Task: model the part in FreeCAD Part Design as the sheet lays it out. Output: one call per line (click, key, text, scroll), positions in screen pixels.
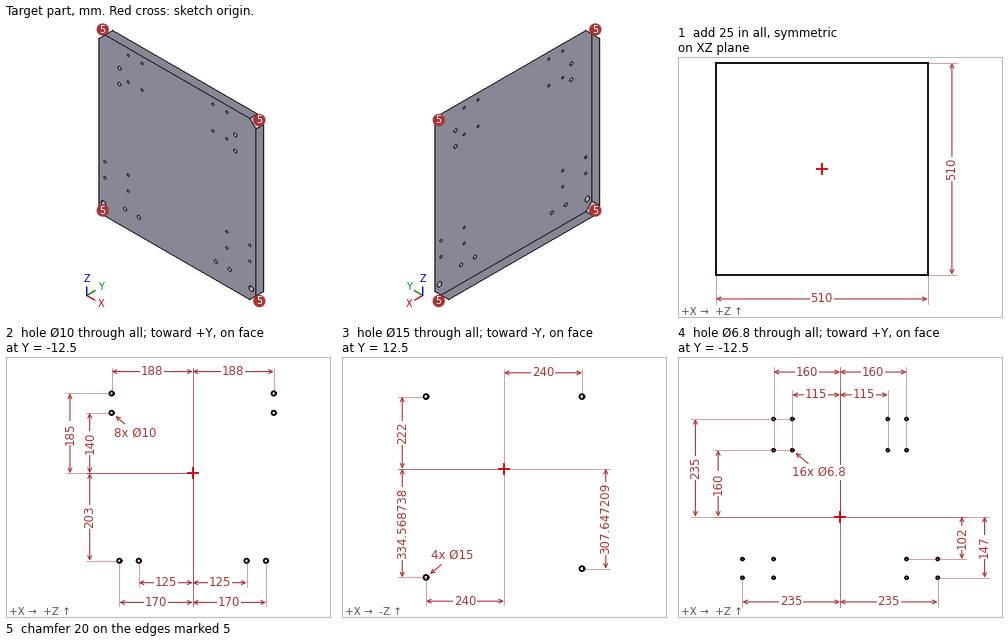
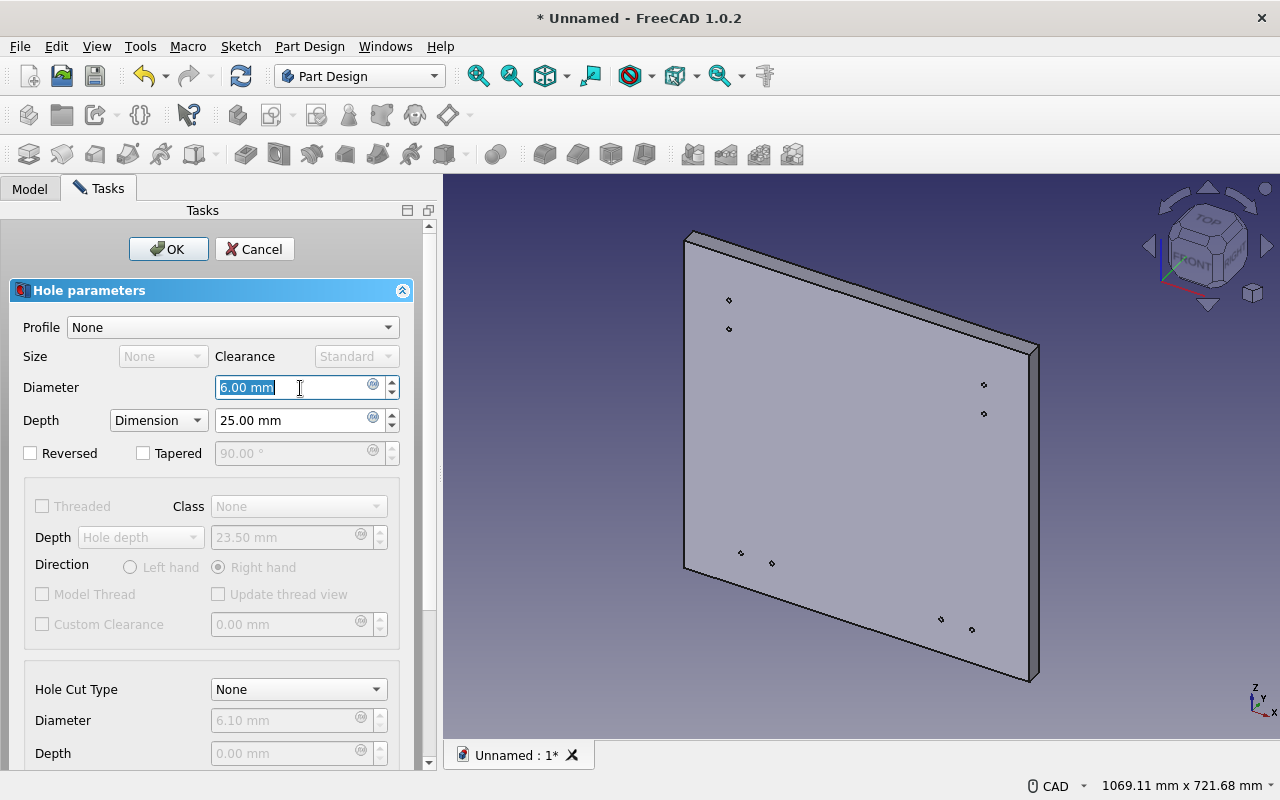
text(10)
key(Tab)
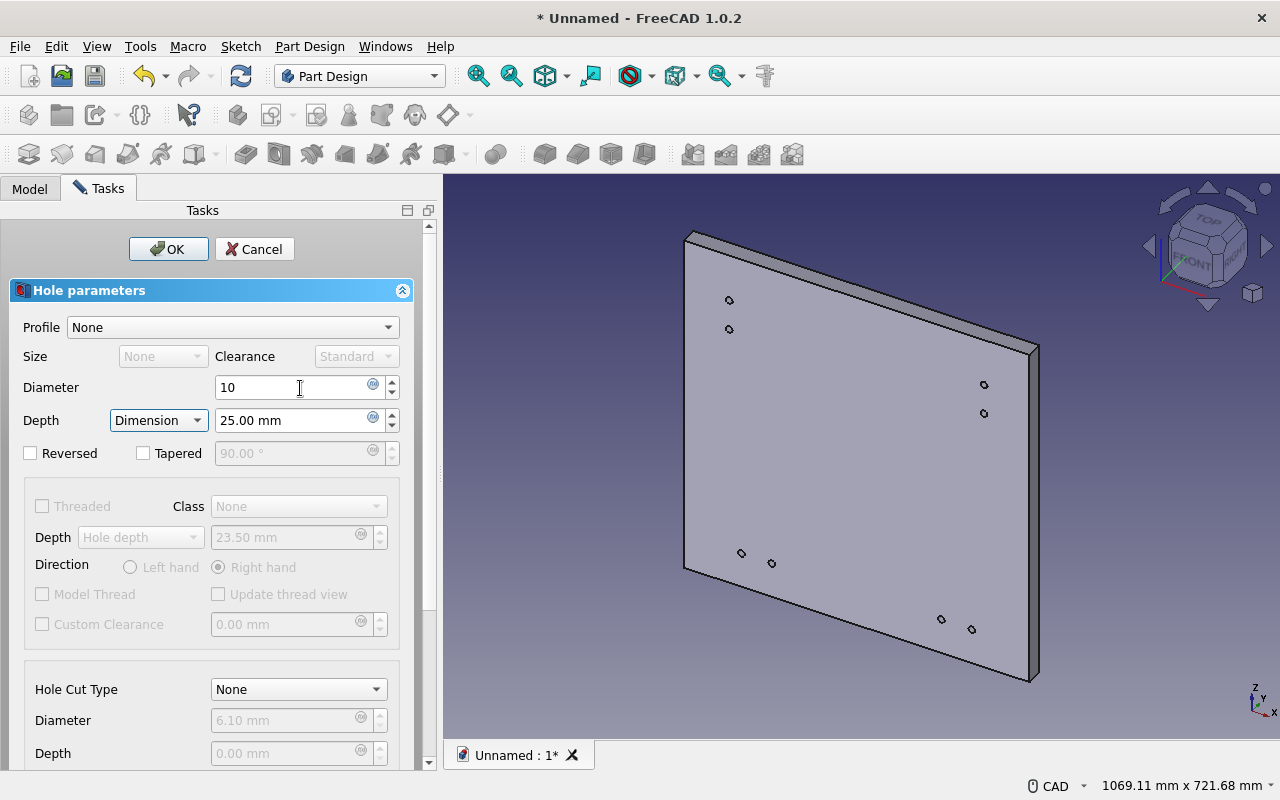
click(160, 420)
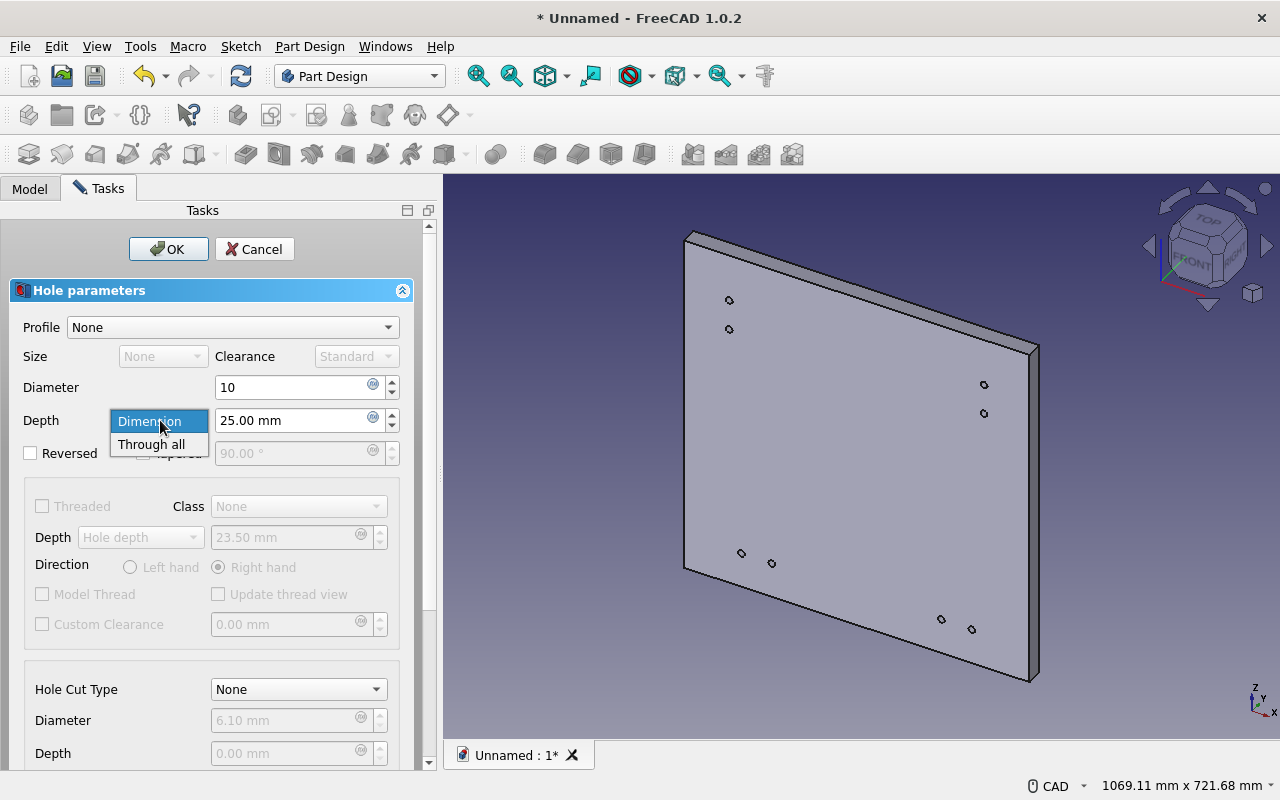
click(158, 444)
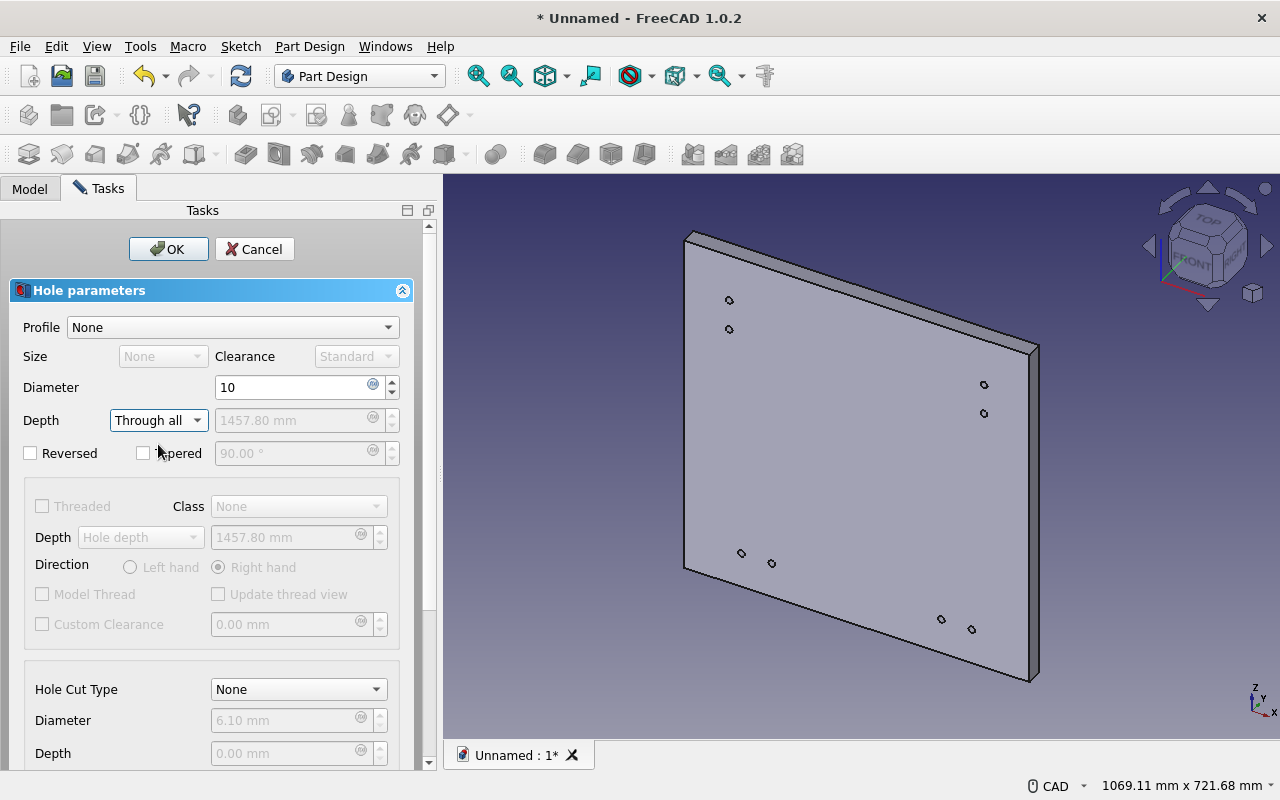
click(169, 249)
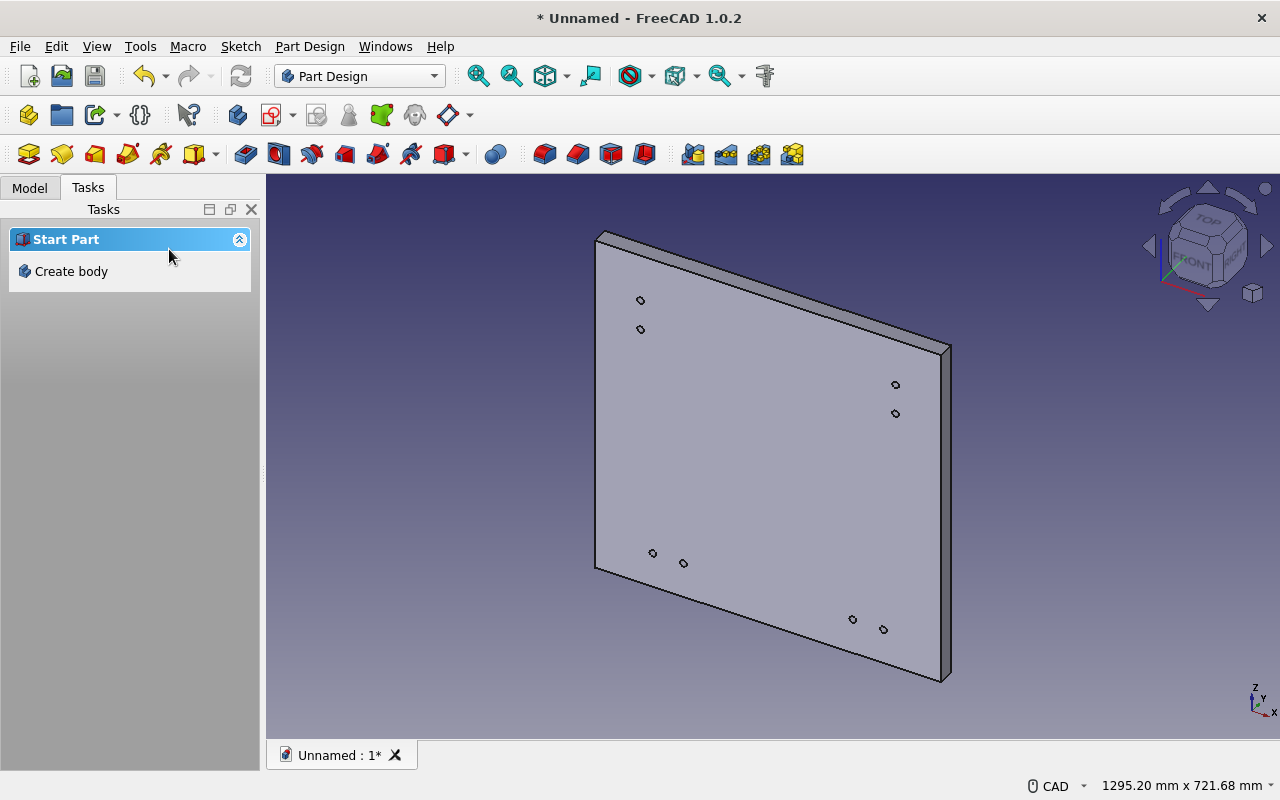
key(4)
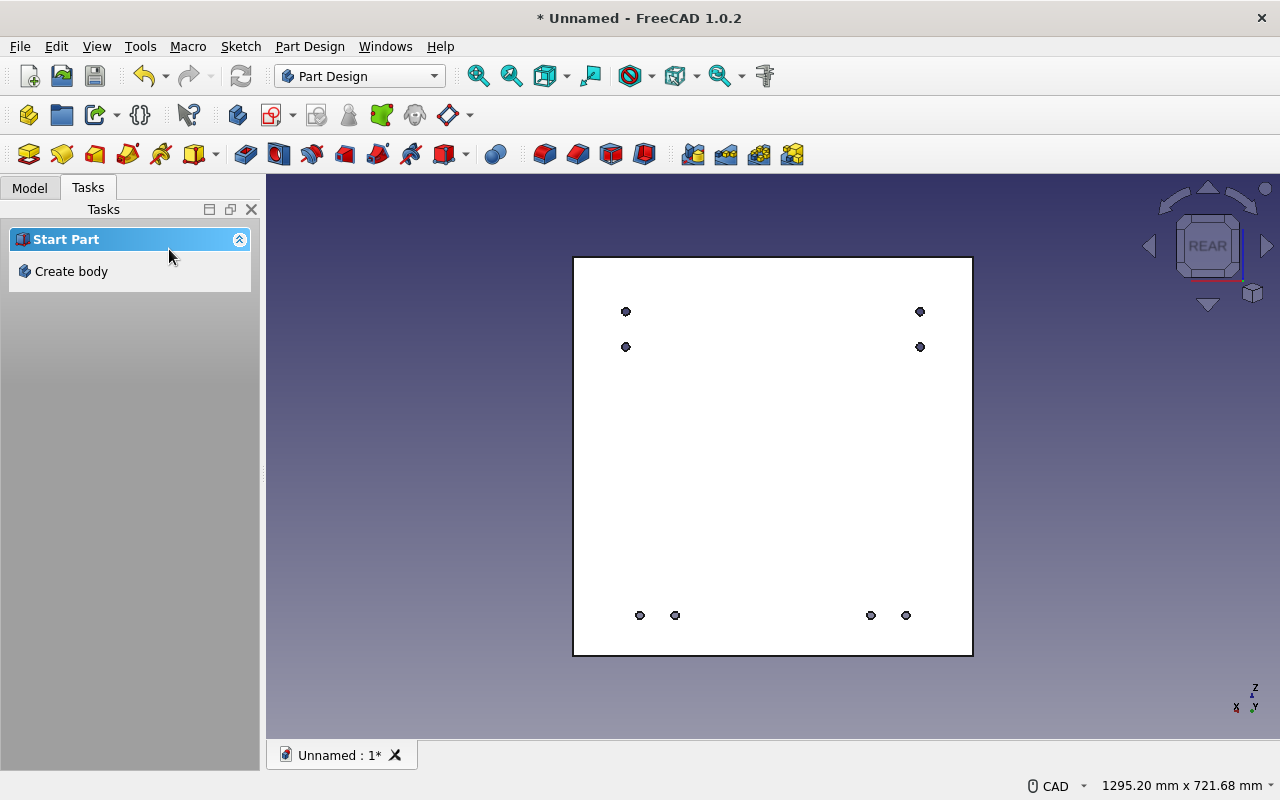
click(773, 456)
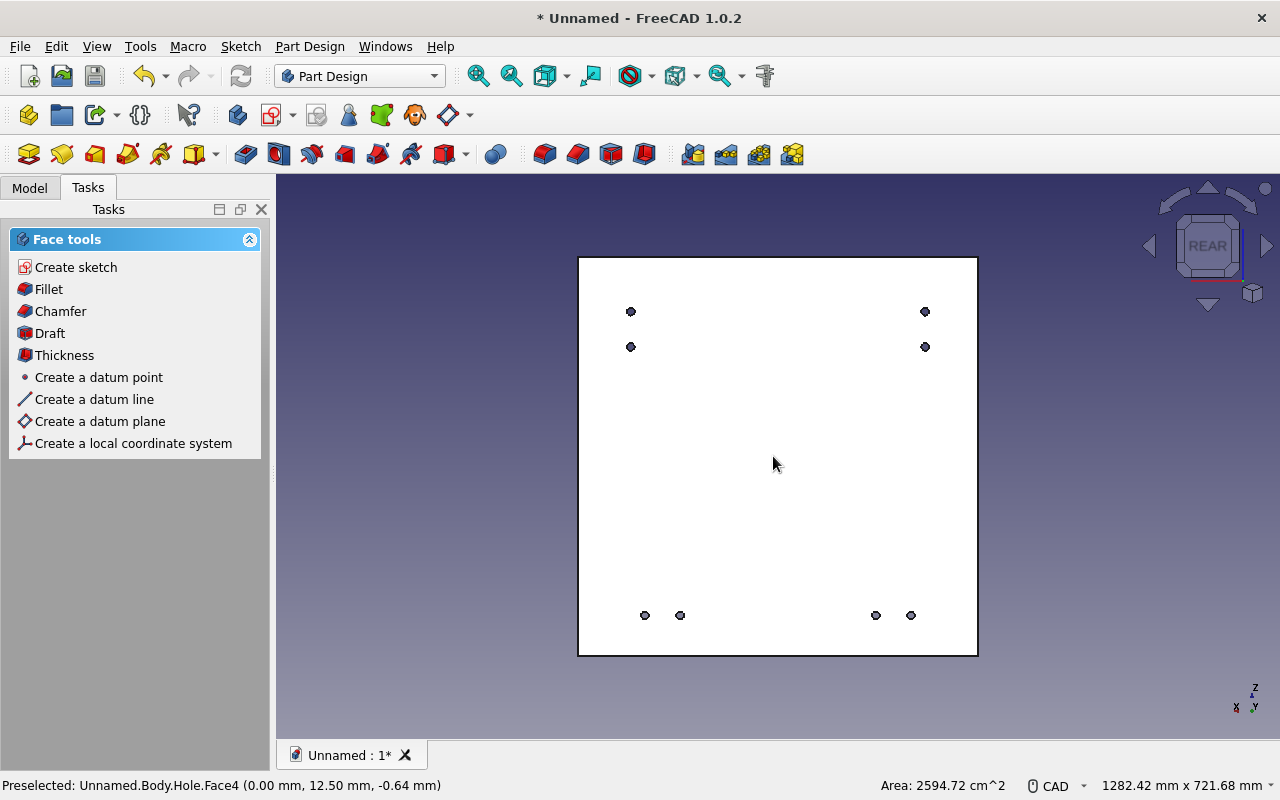
click(270, 116)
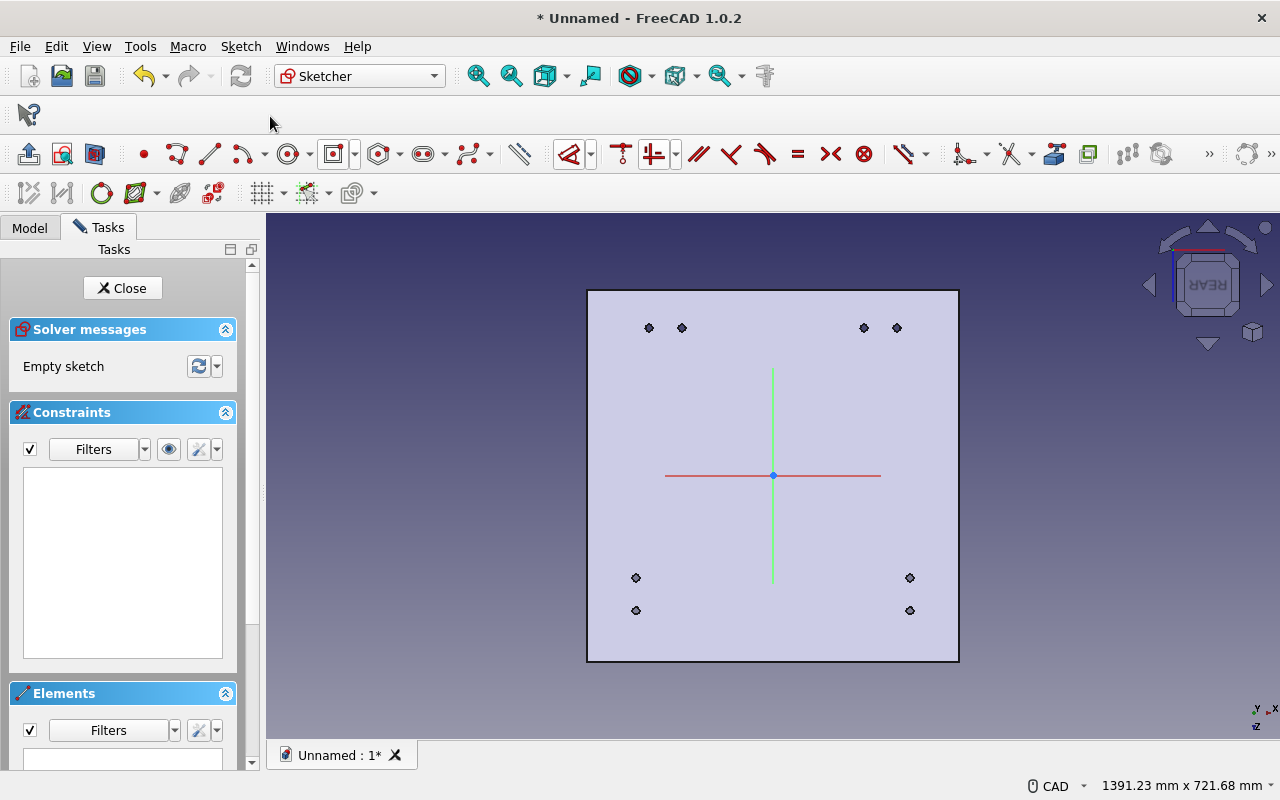
scroll(395, 291, down, 1)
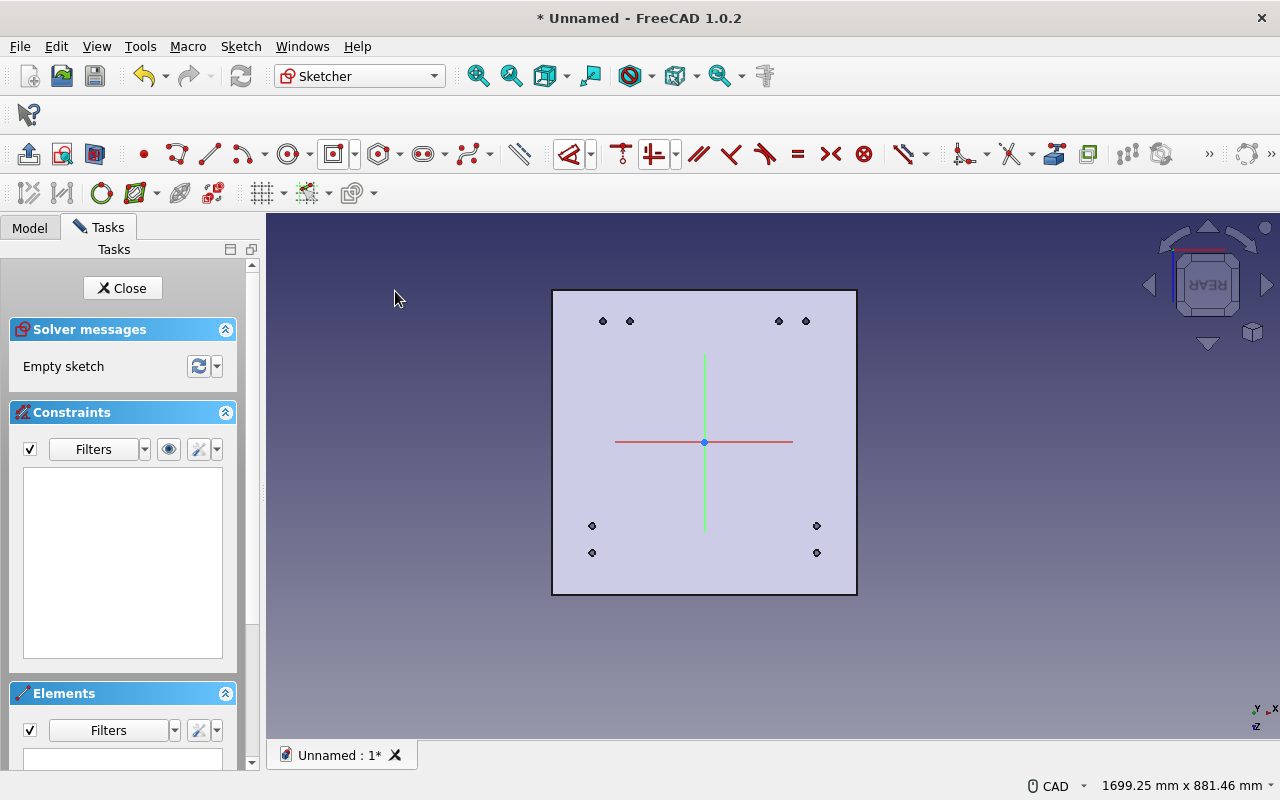
click(288, 154)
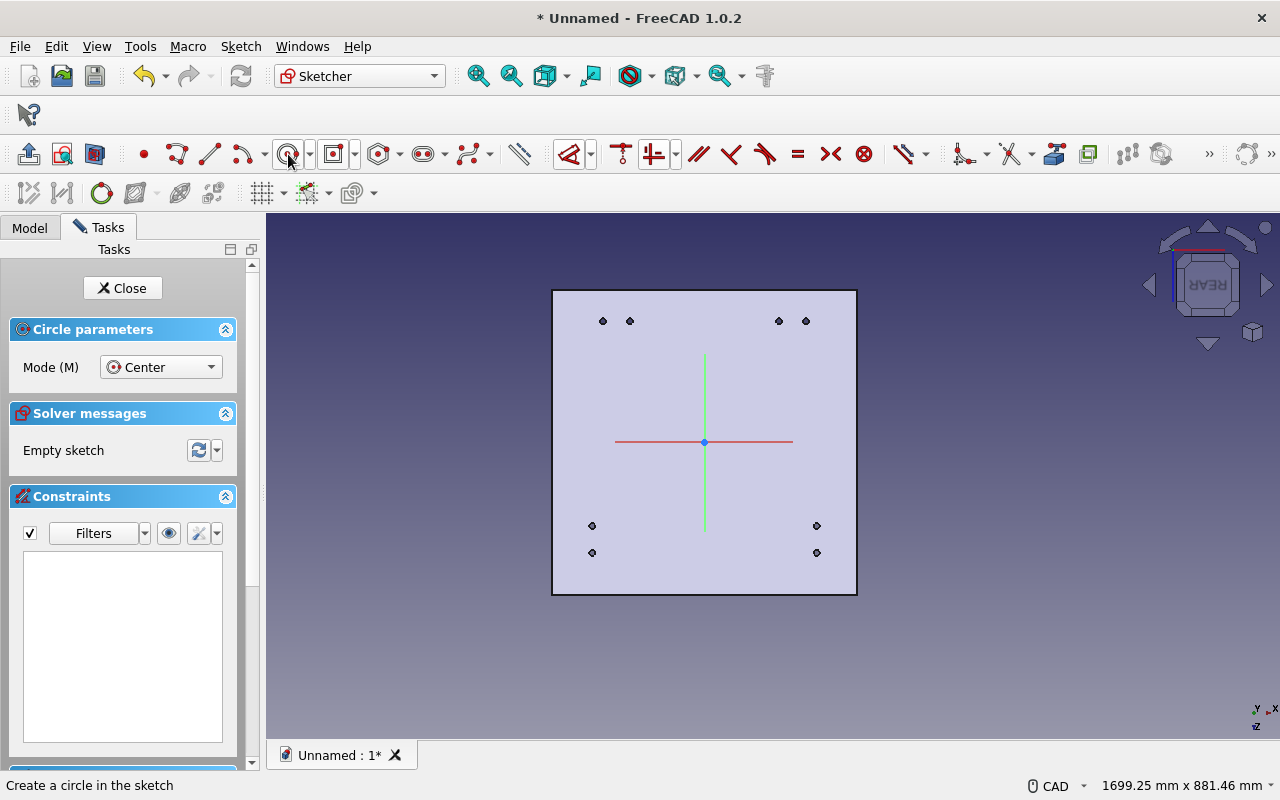
scroll(561, 642, up, 9)